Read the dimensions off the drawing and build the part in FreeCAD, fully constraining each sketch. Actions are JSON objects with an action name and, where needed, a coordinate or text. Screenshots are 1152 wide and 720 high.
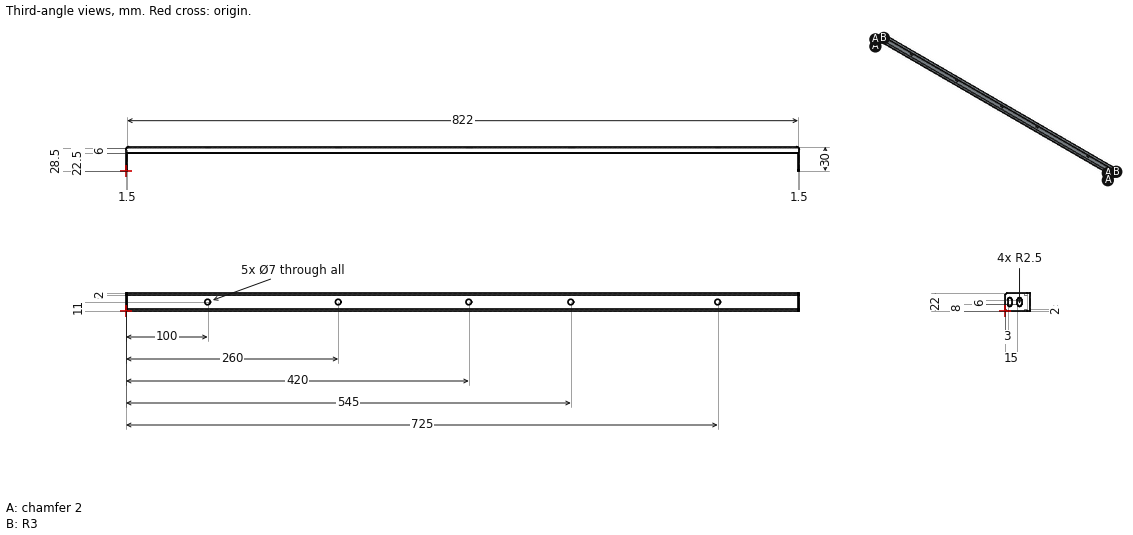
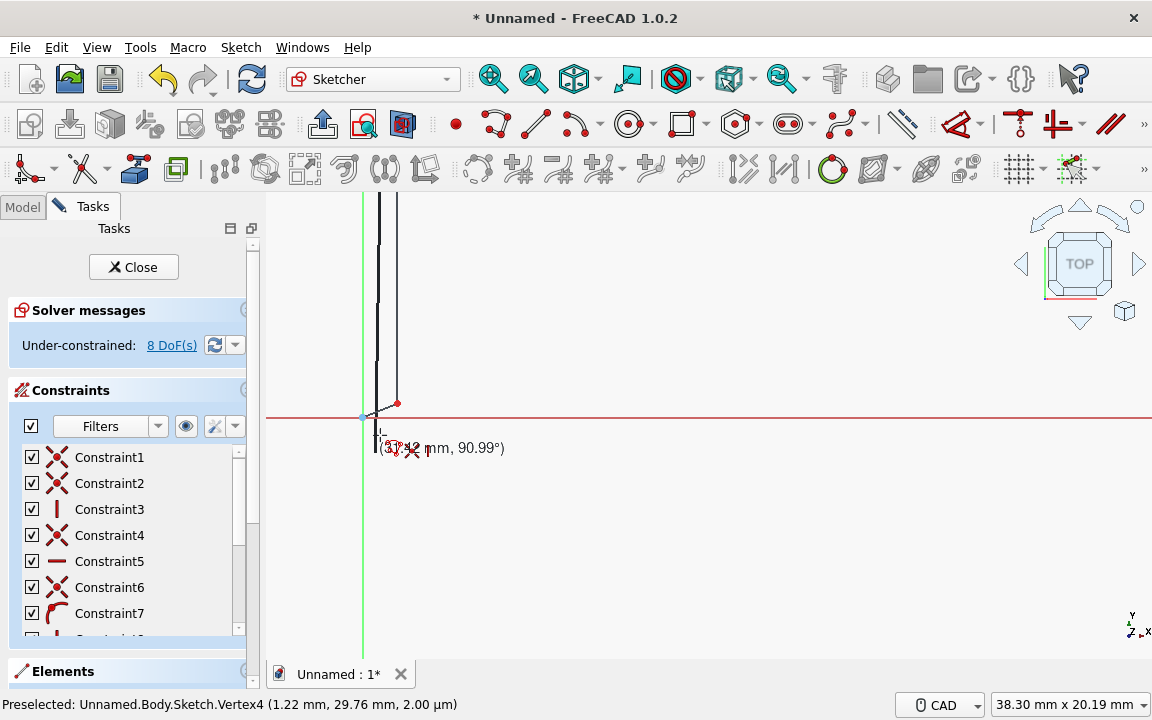
{"action": "left_click", "coordinate": [363, 418]}
{"action": "key", "text": "Escape"}
{"action": "key", "text": "Escape"}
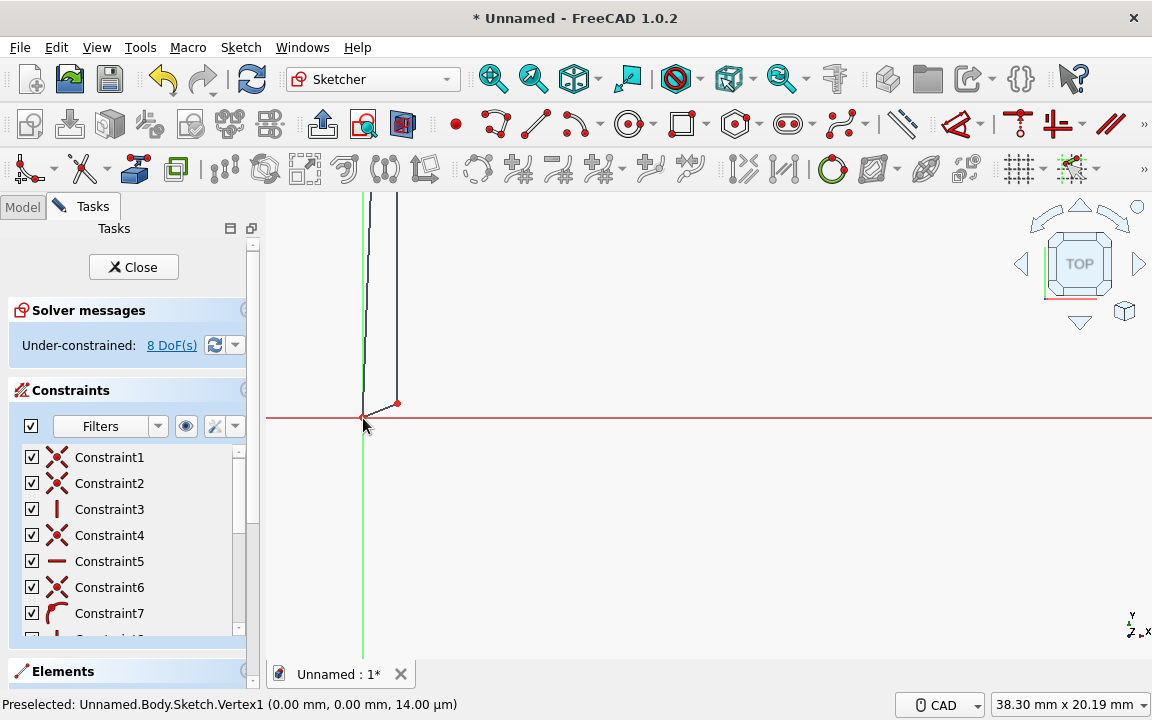
{"action": "left_click", "coordinate": [387, 408]}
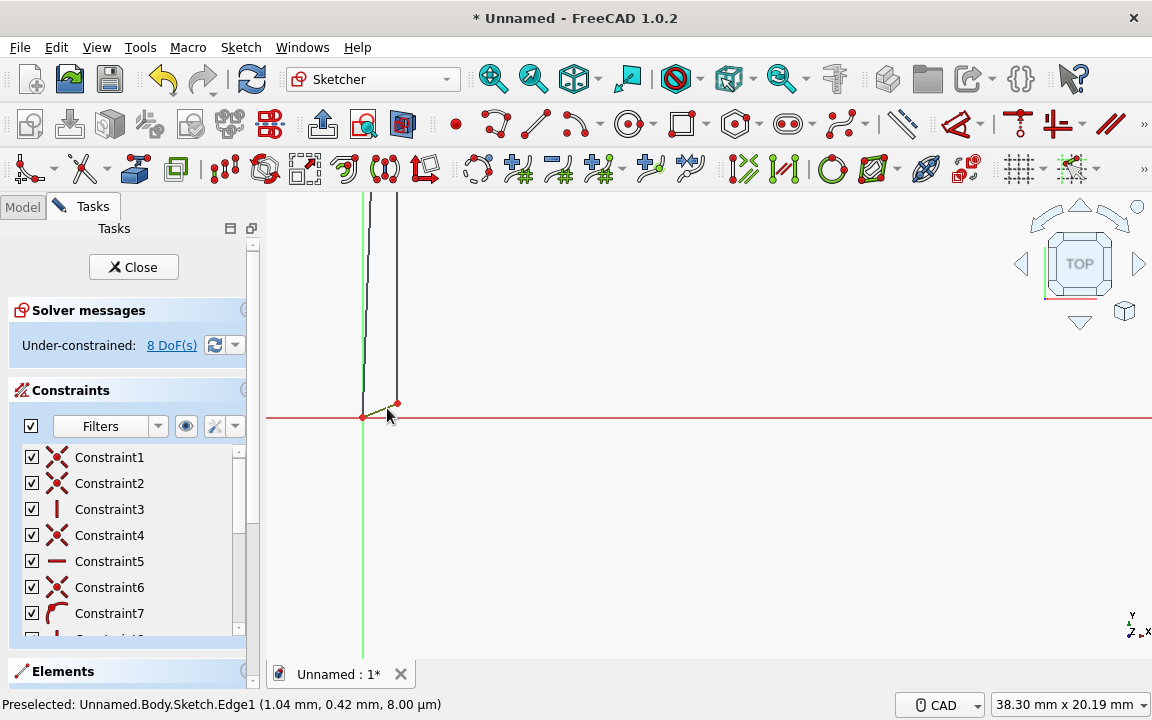
{"action": "left_click", "coordinate": [1084, 124]}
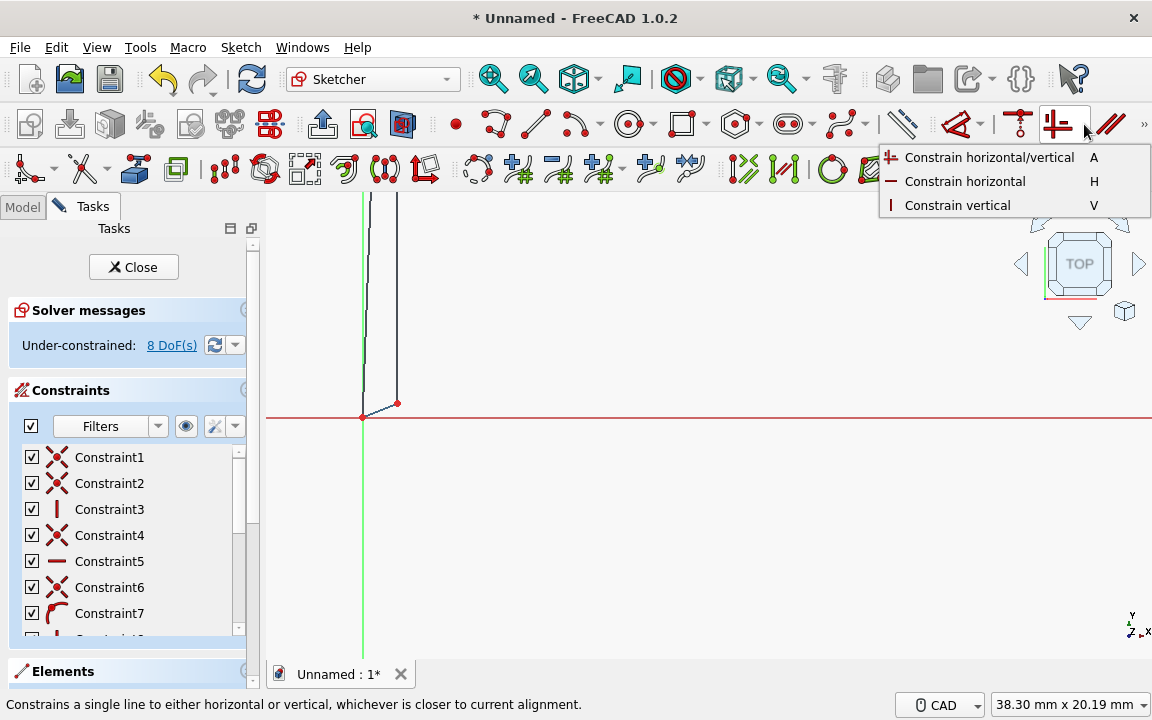
{"action": "left_click", "coordinate": [1015, 181]}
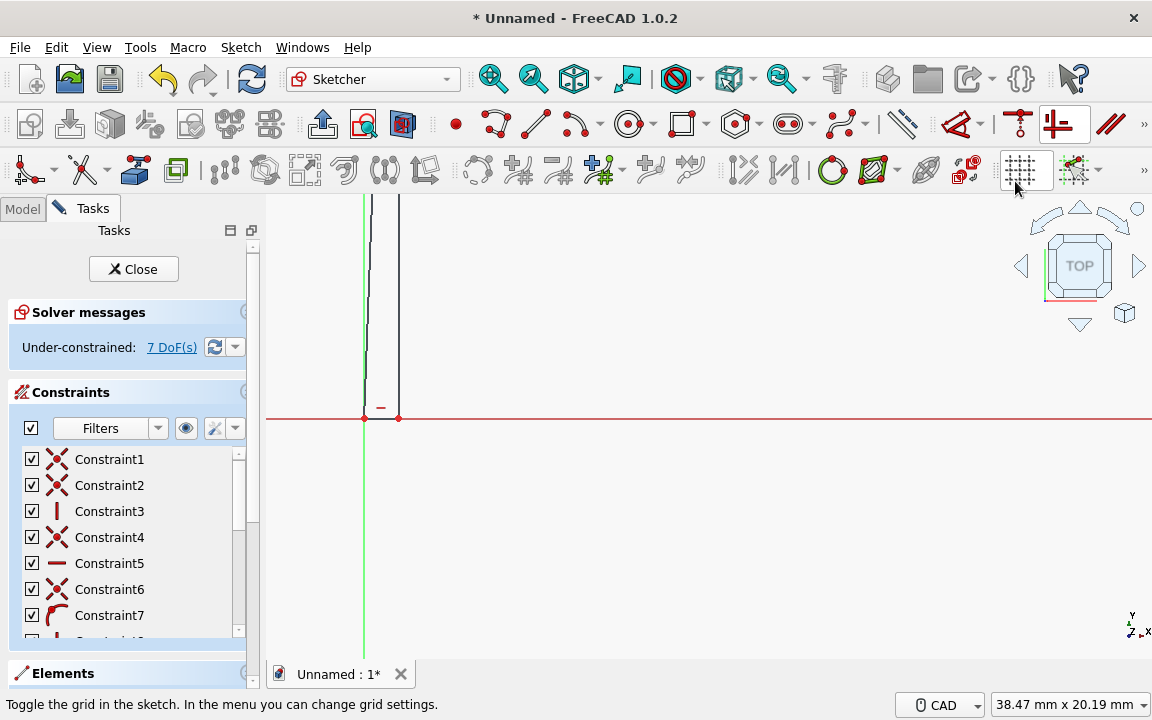
{"action": "scroll", "coordinate": [322, 439], "scroll_direction": "down", "scroll_amount": 17}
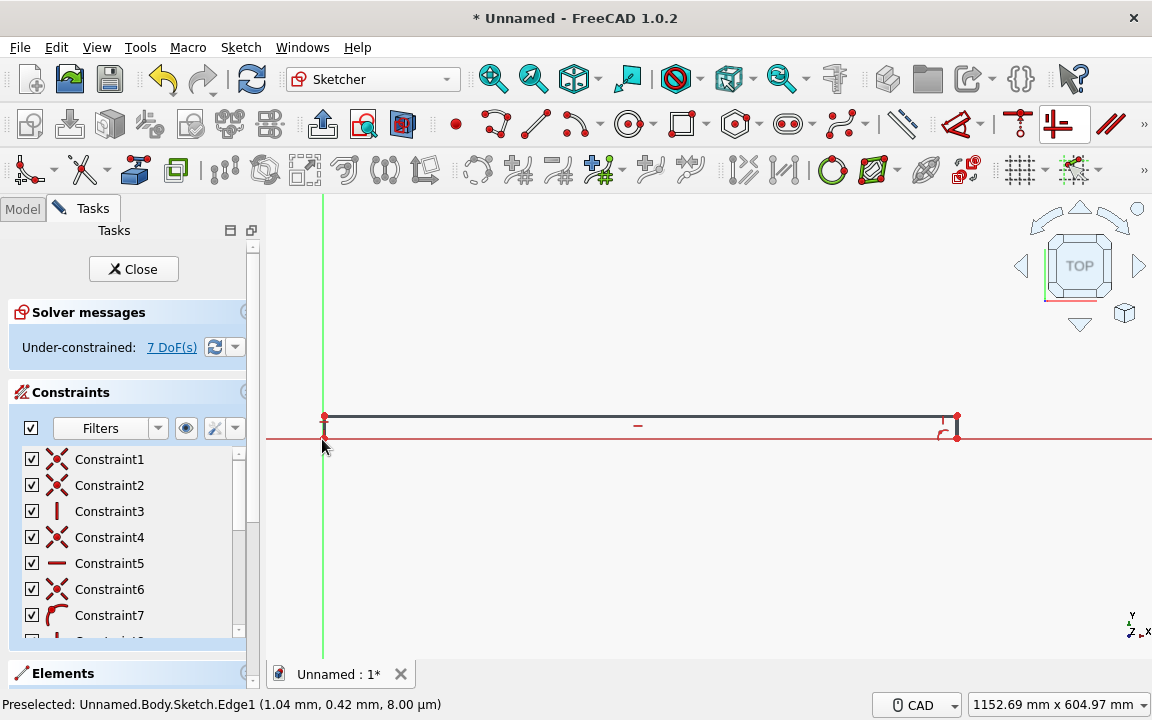
{"action": "scroll", "coordinate": [957, 439], "scroll_direction": "up", "scroll_amount": 13}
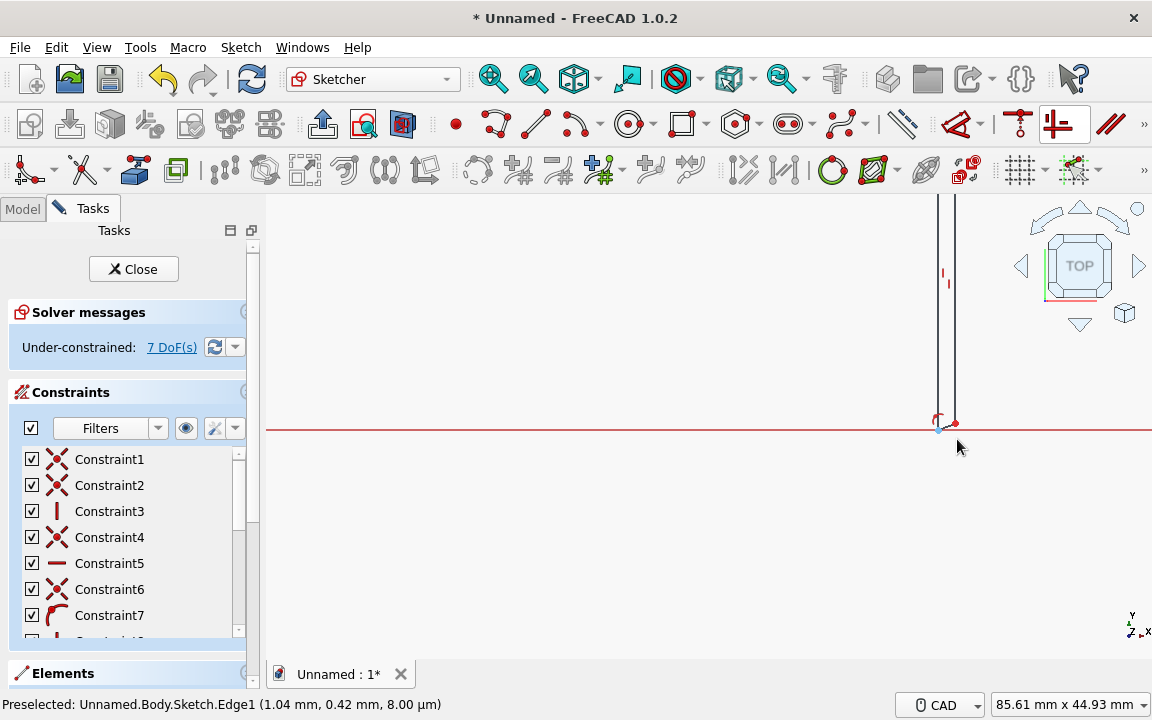
{"action": "left_click", "coordinate": [950, 426]}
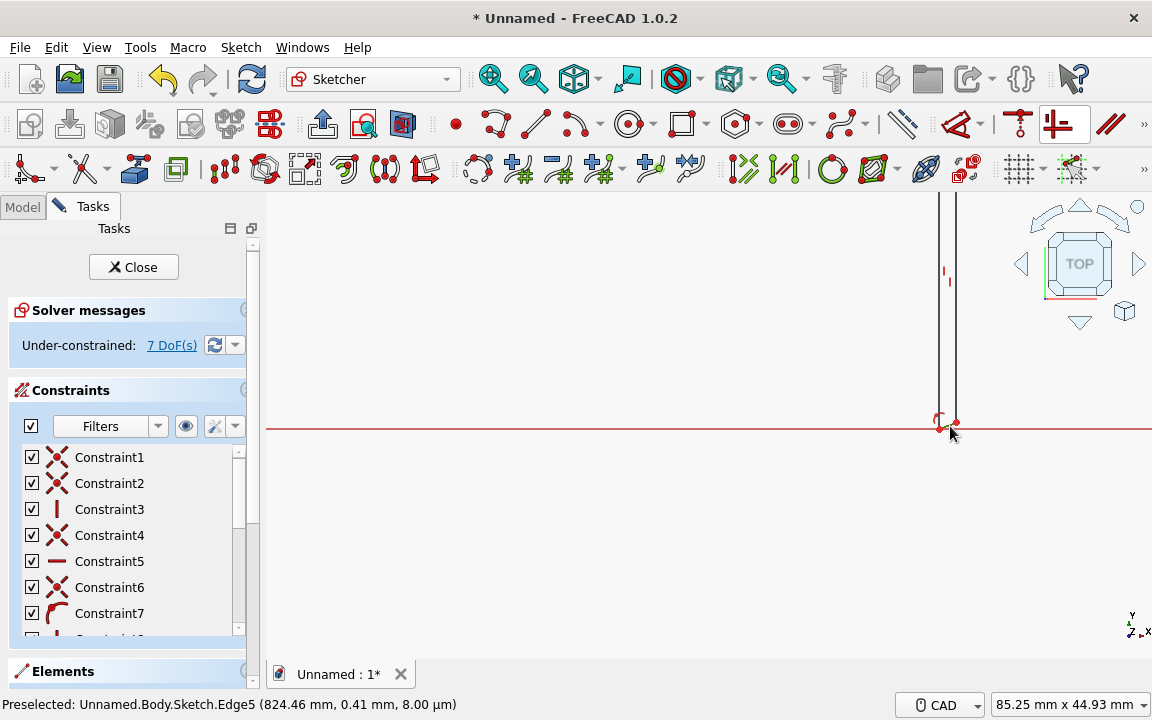
{"action": "left_click", "coordinate": [1084, 124]}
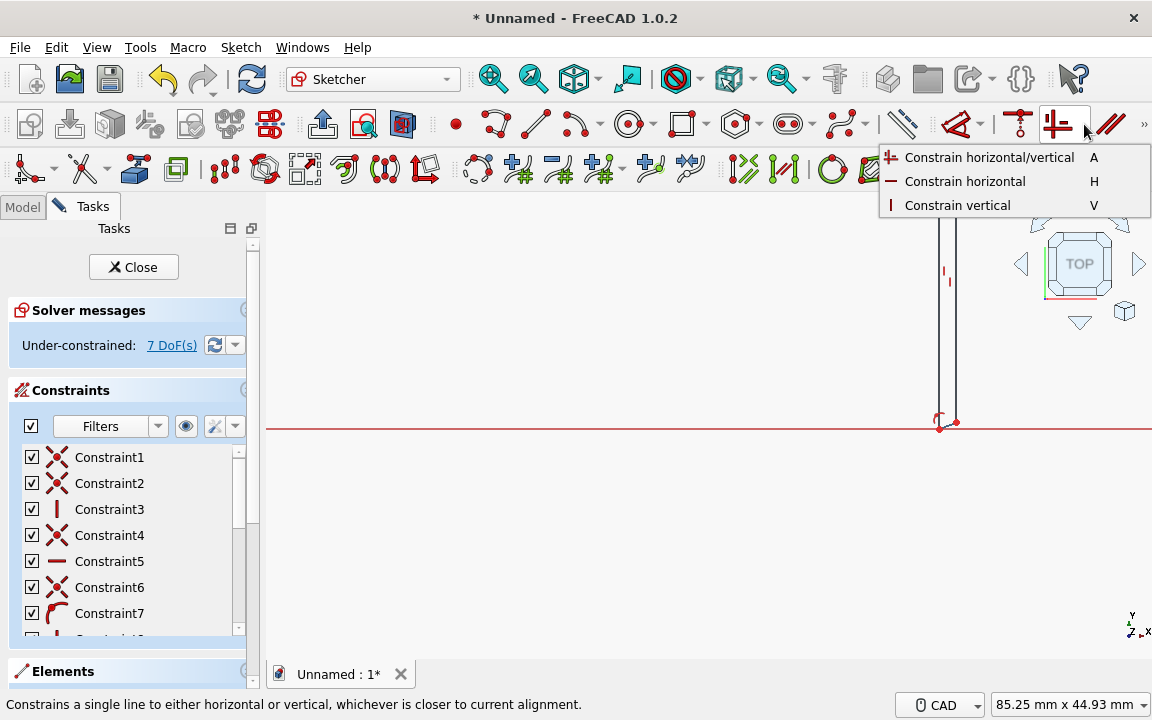
{"action": "left_click", "coordinate": [1015, 181]}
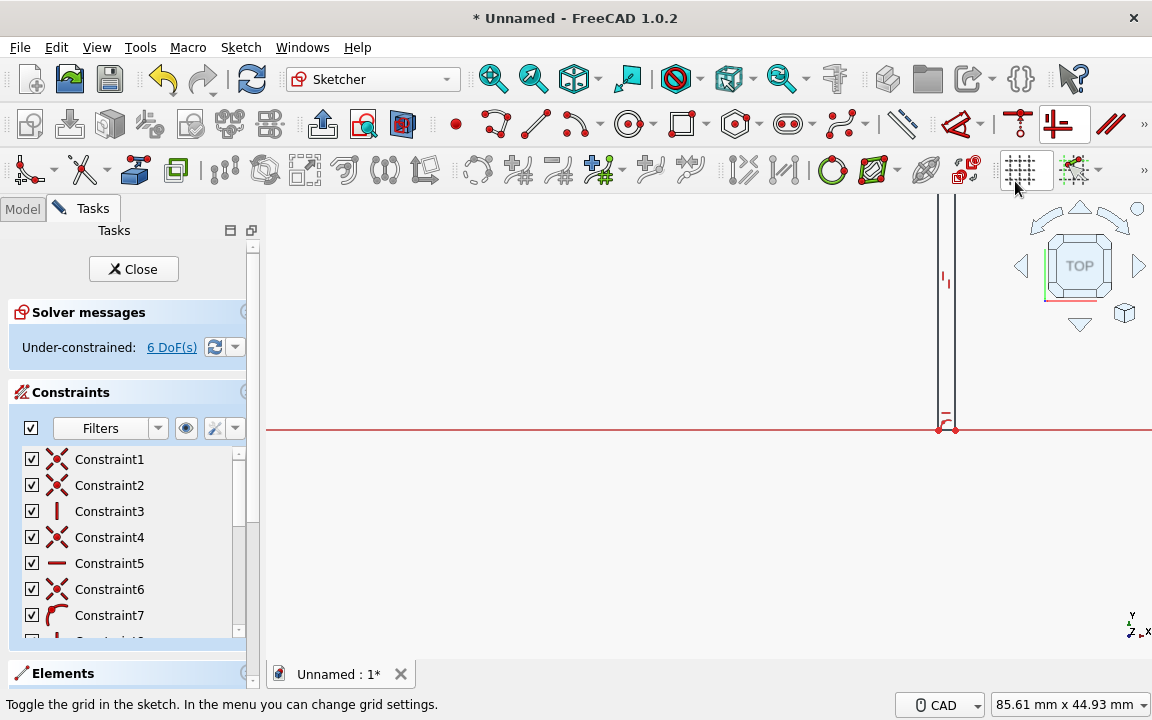
{"action": "scroll", "coordinate": [897, 436], "scroll_direction": "down", "scroll_amount": 14}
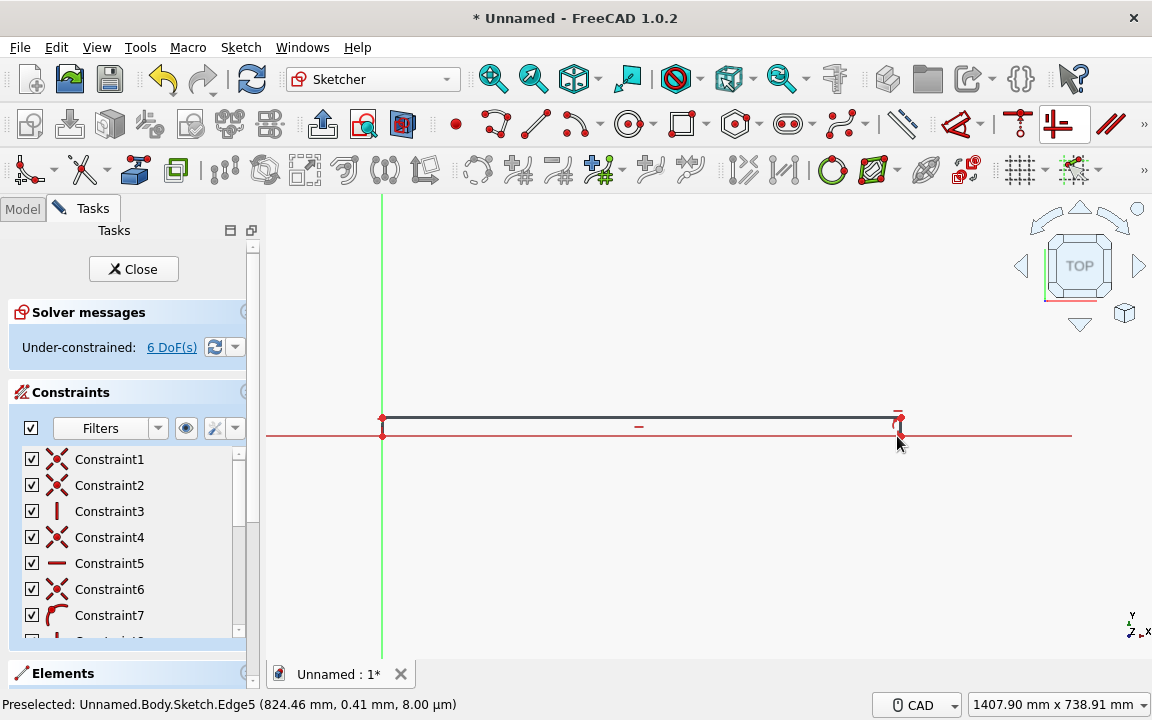
{"action": "scroll", "coordinate": [382, 430], "scroll_direction": "up", "scroll_amount": 14}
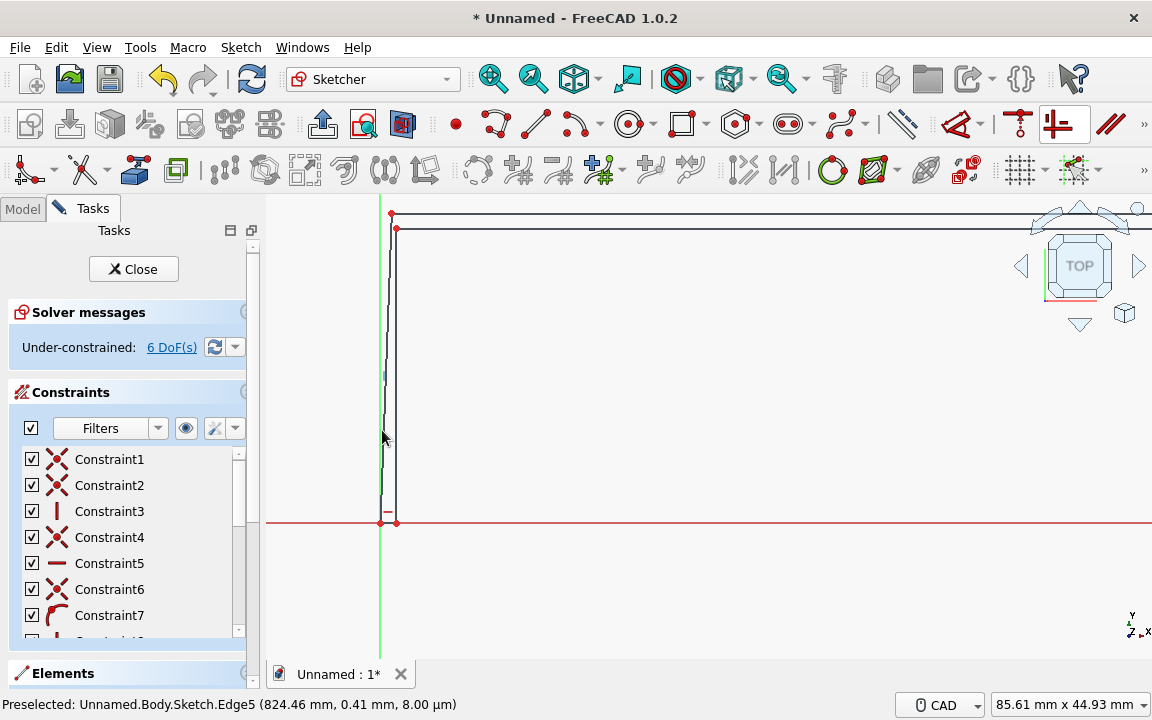
{"action": "left_click", "coordinate": [384, 430]}